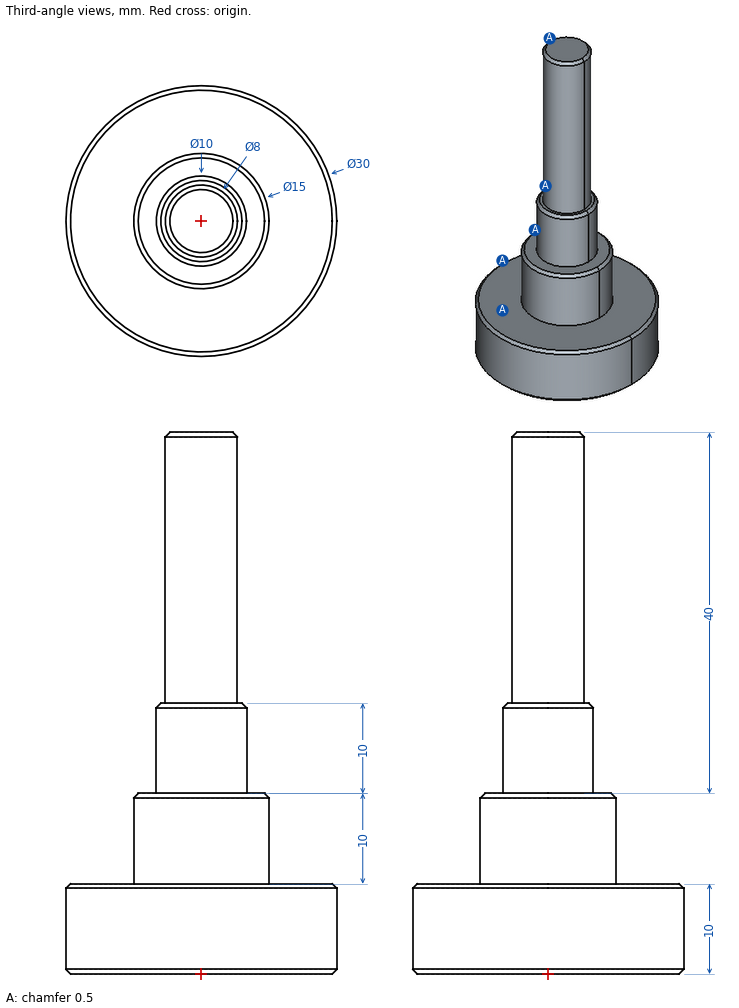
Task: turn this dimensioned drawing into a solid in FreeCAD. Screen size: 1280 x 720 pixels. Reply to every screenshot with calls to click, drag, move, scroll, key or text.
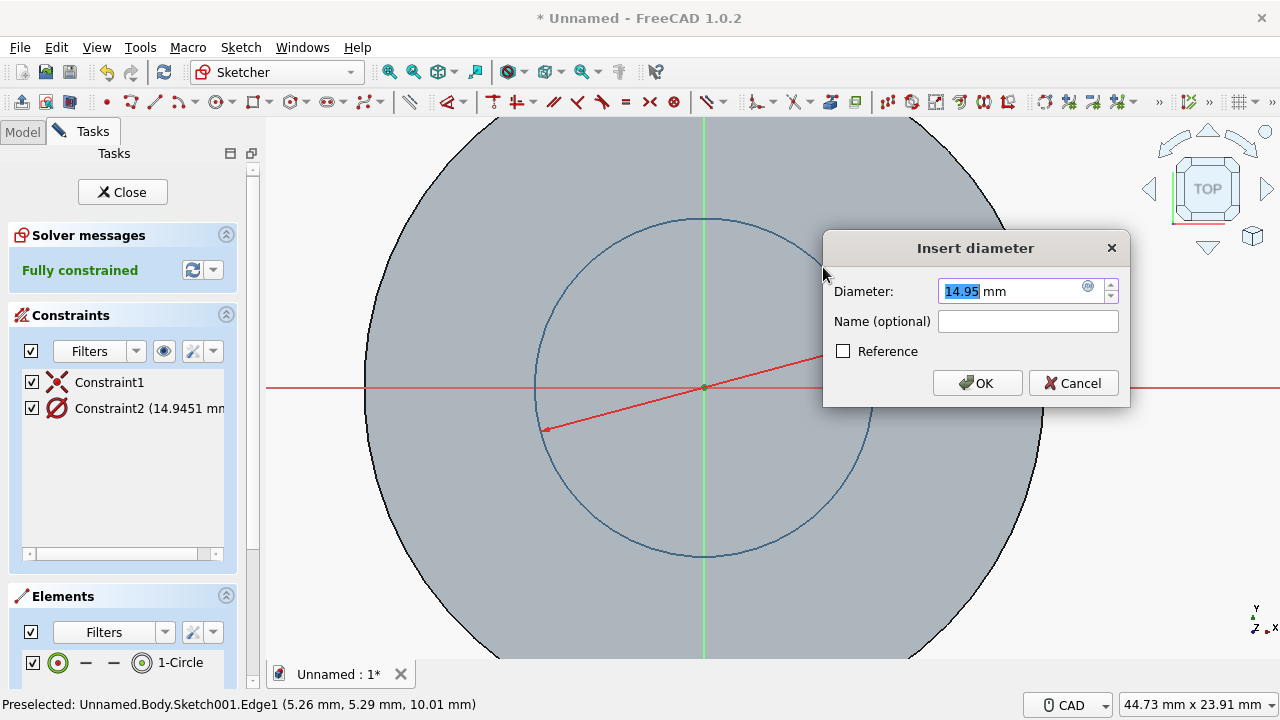
text(15)
key(Return)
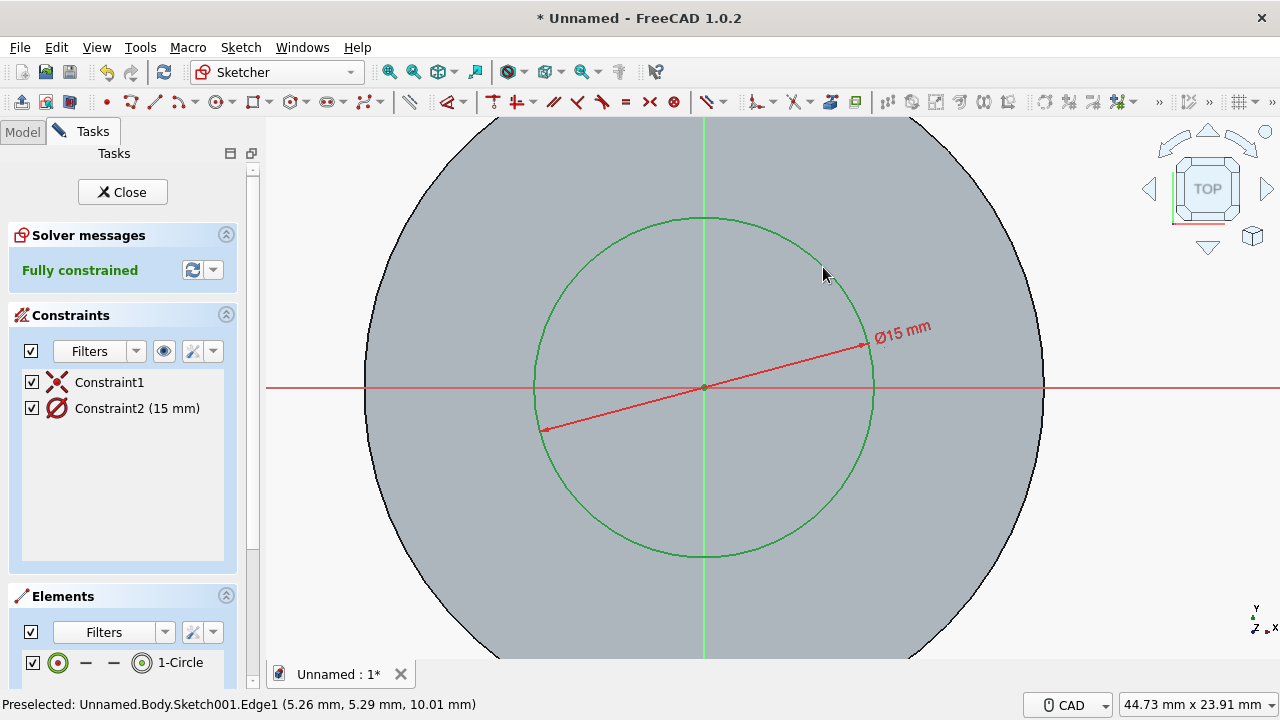
click(123, 192)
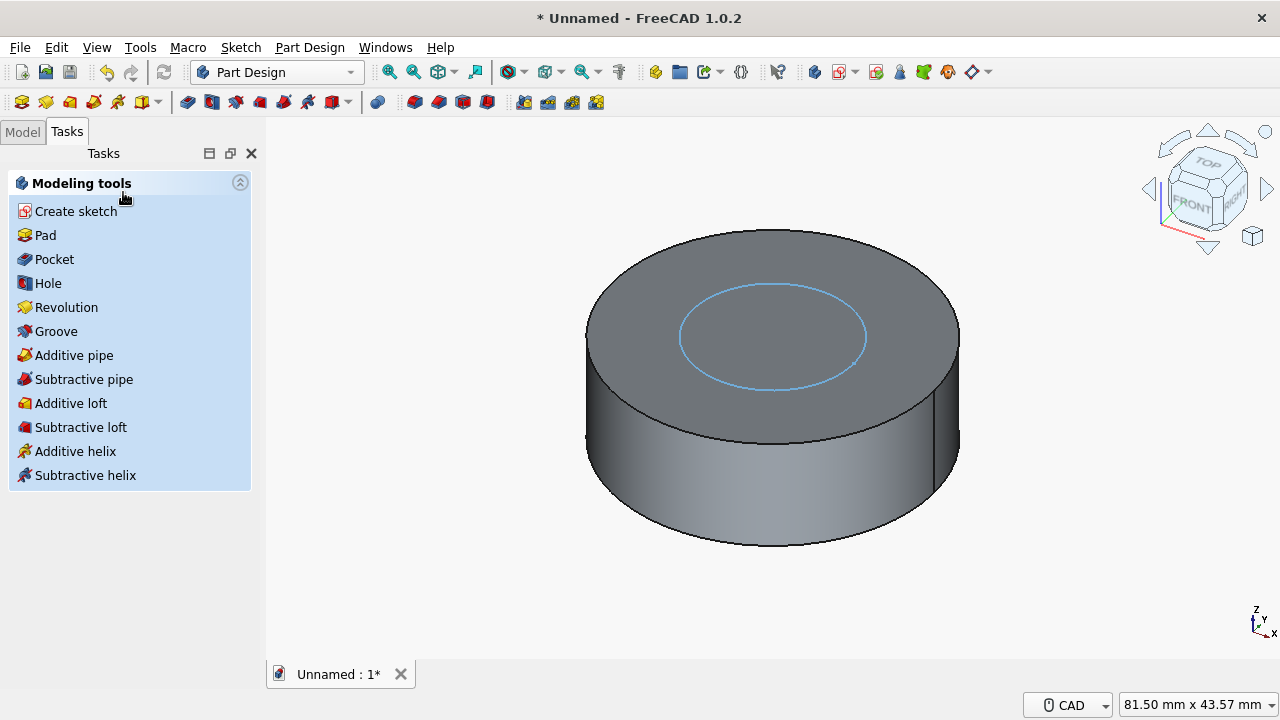
click(22, 102)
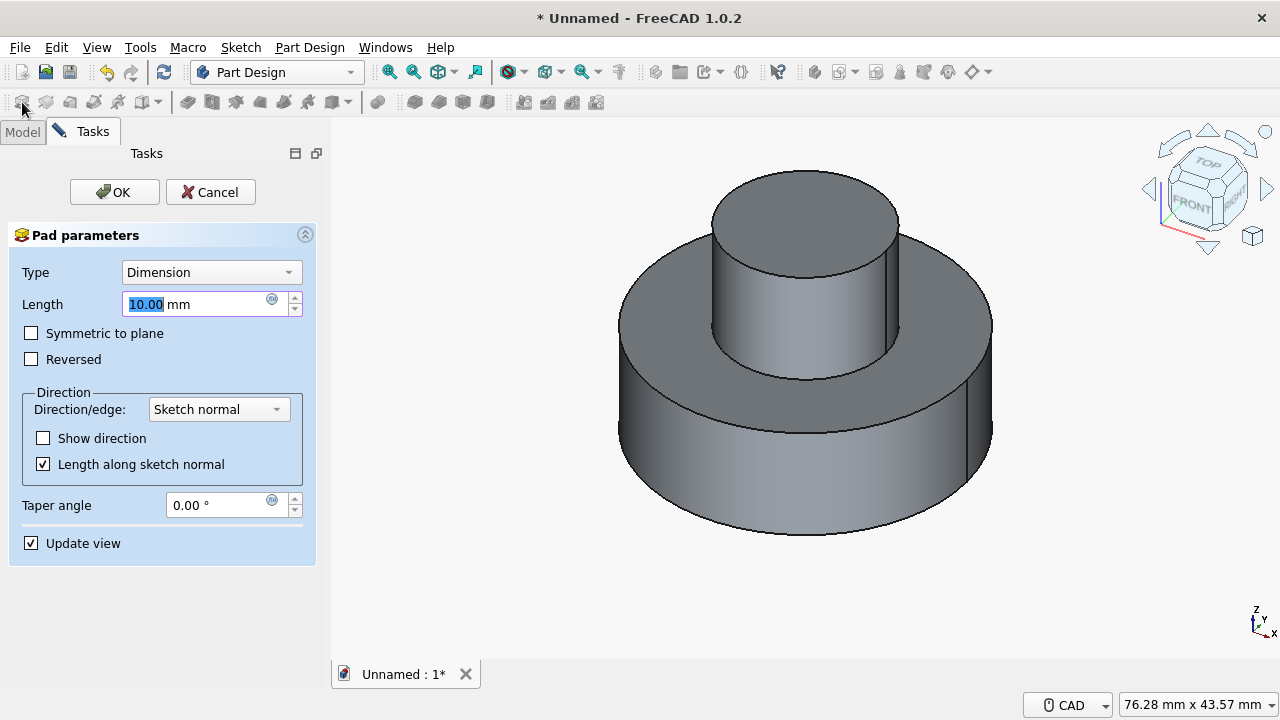
text(10)
key(Tab)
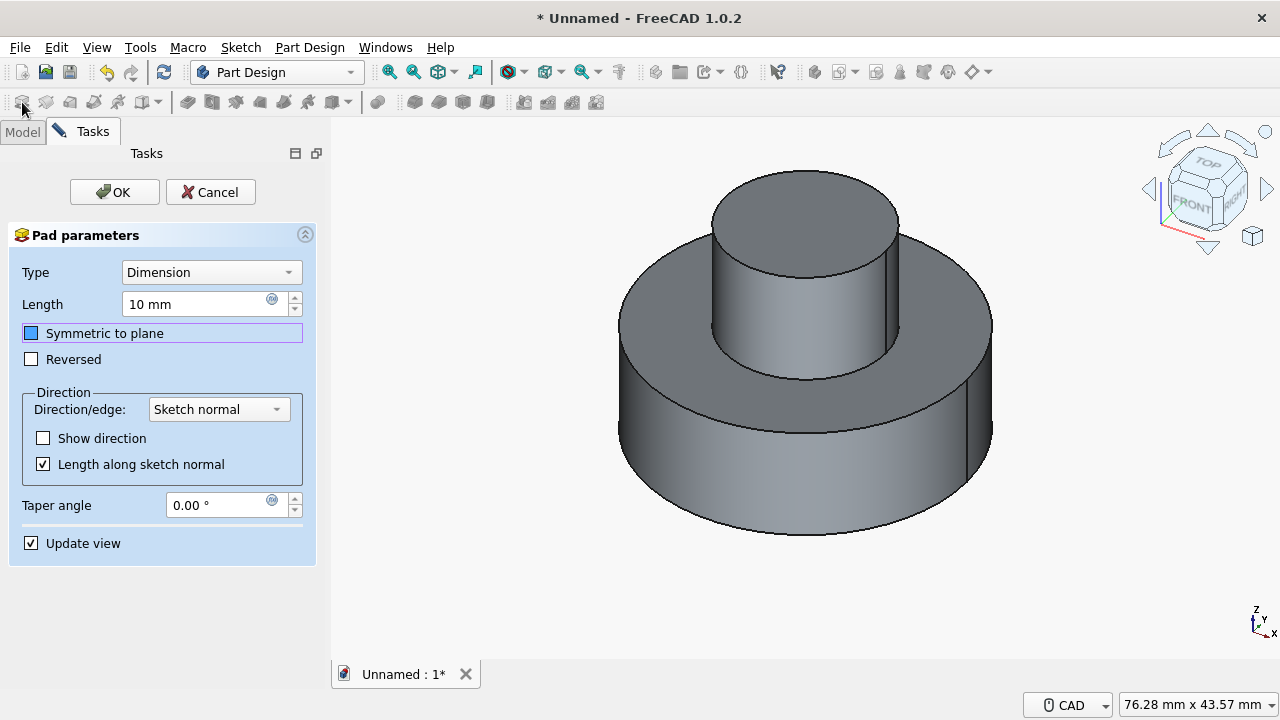
click(115, 192)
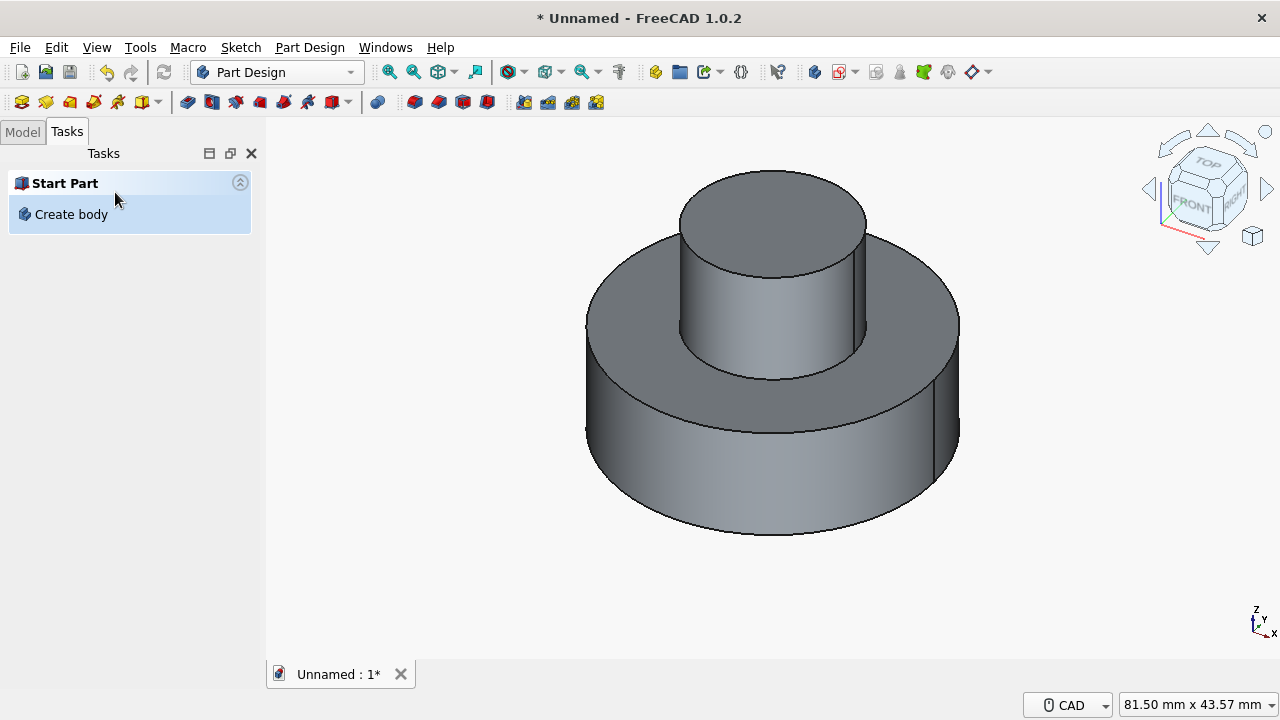
key(v)
key(f)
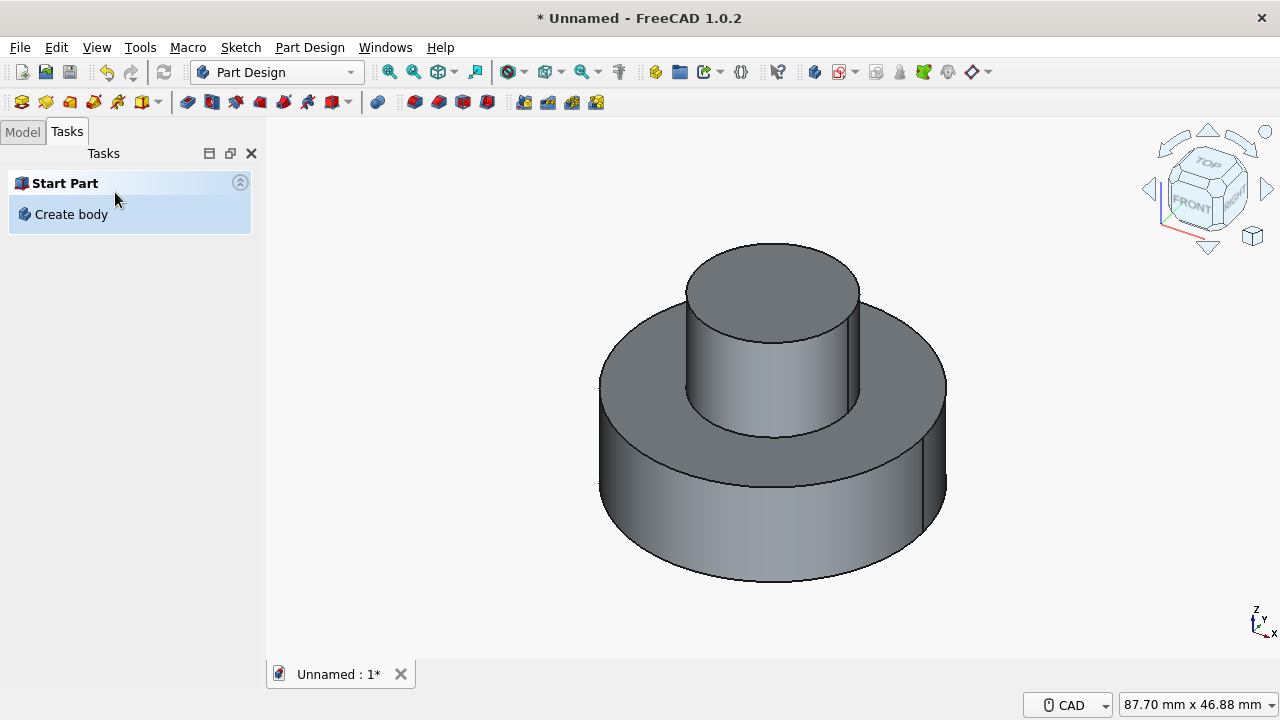
click(773, 292)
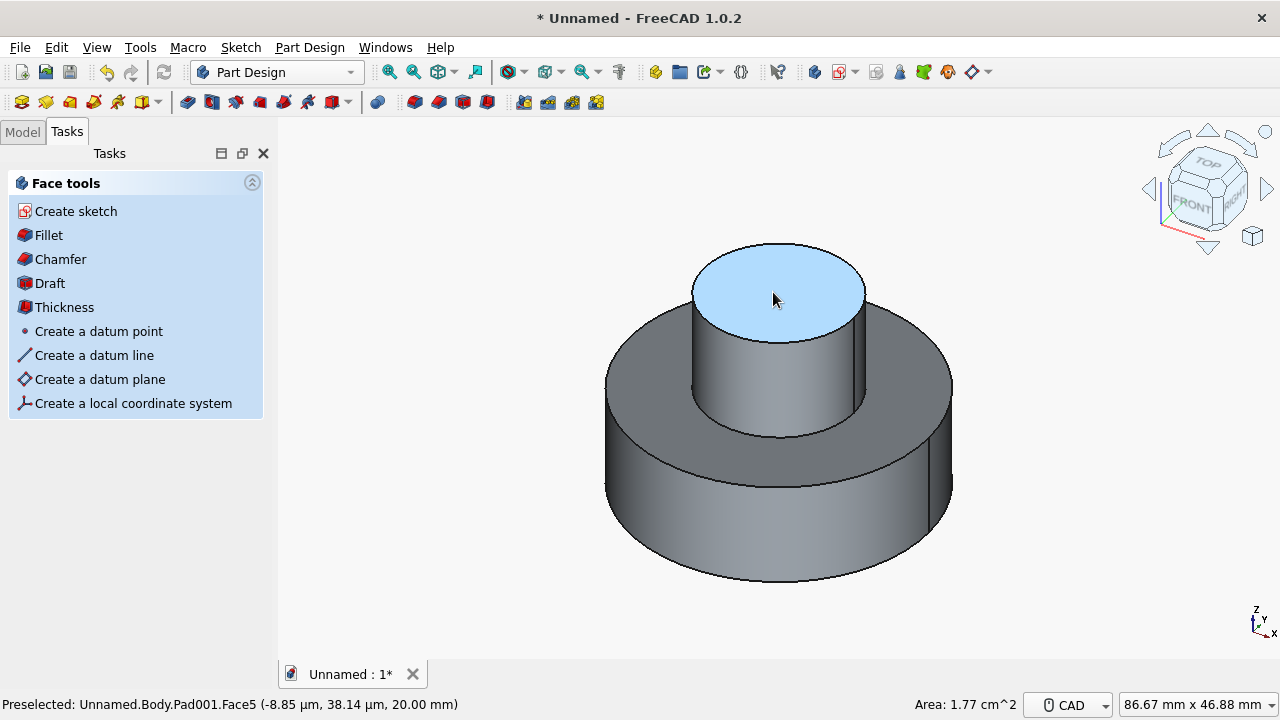
click(840, 72)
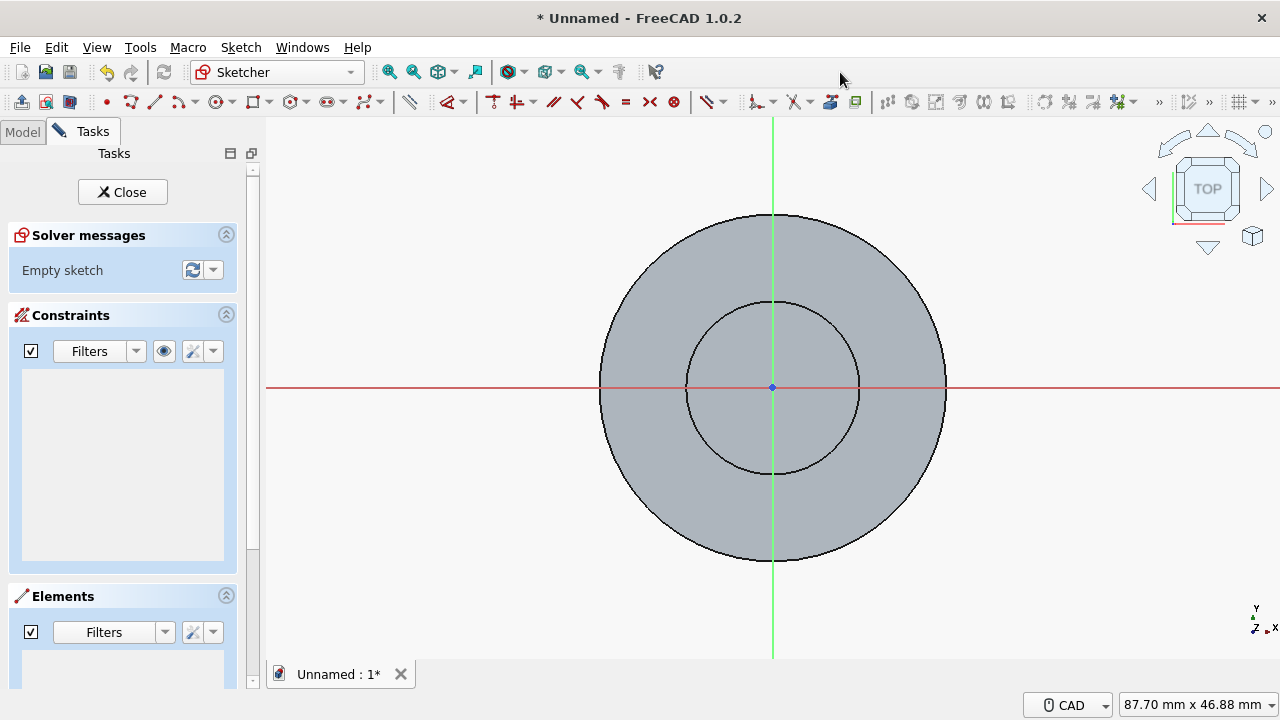
scroll(795, 388, up, 7)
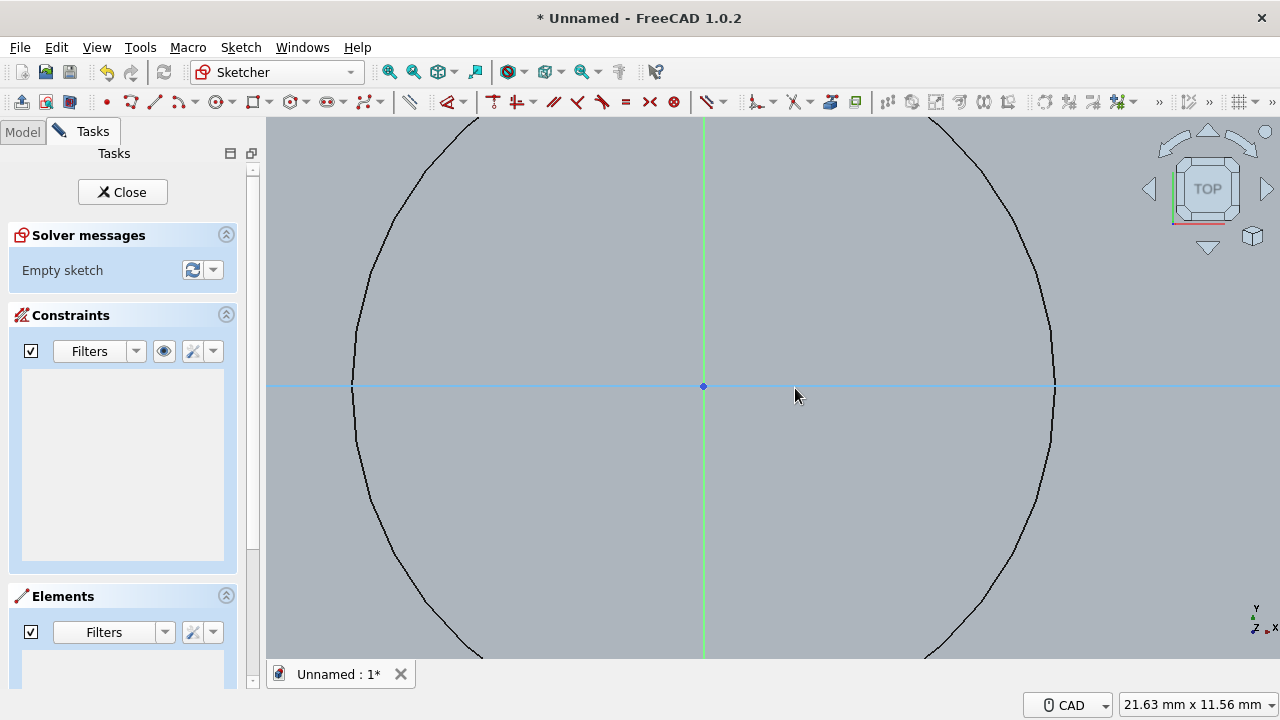
click(216, 102)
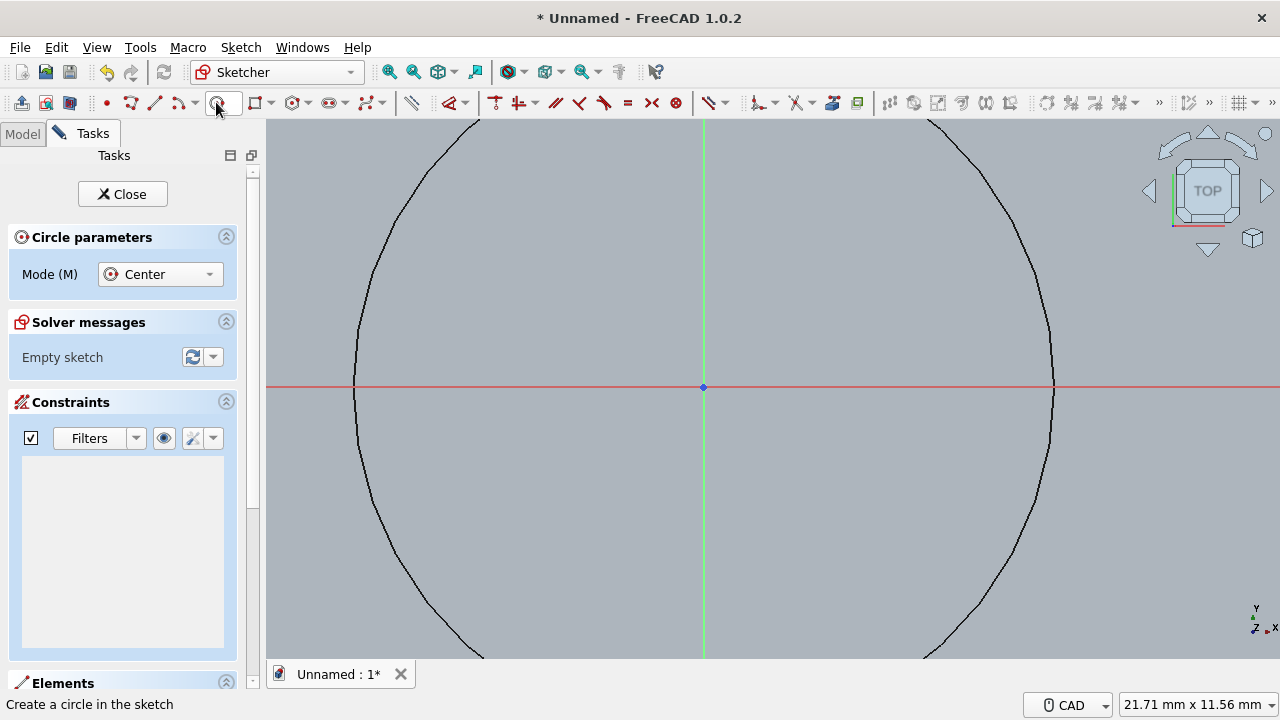
click(704, 387)
click(836, 255)
key(Escape)